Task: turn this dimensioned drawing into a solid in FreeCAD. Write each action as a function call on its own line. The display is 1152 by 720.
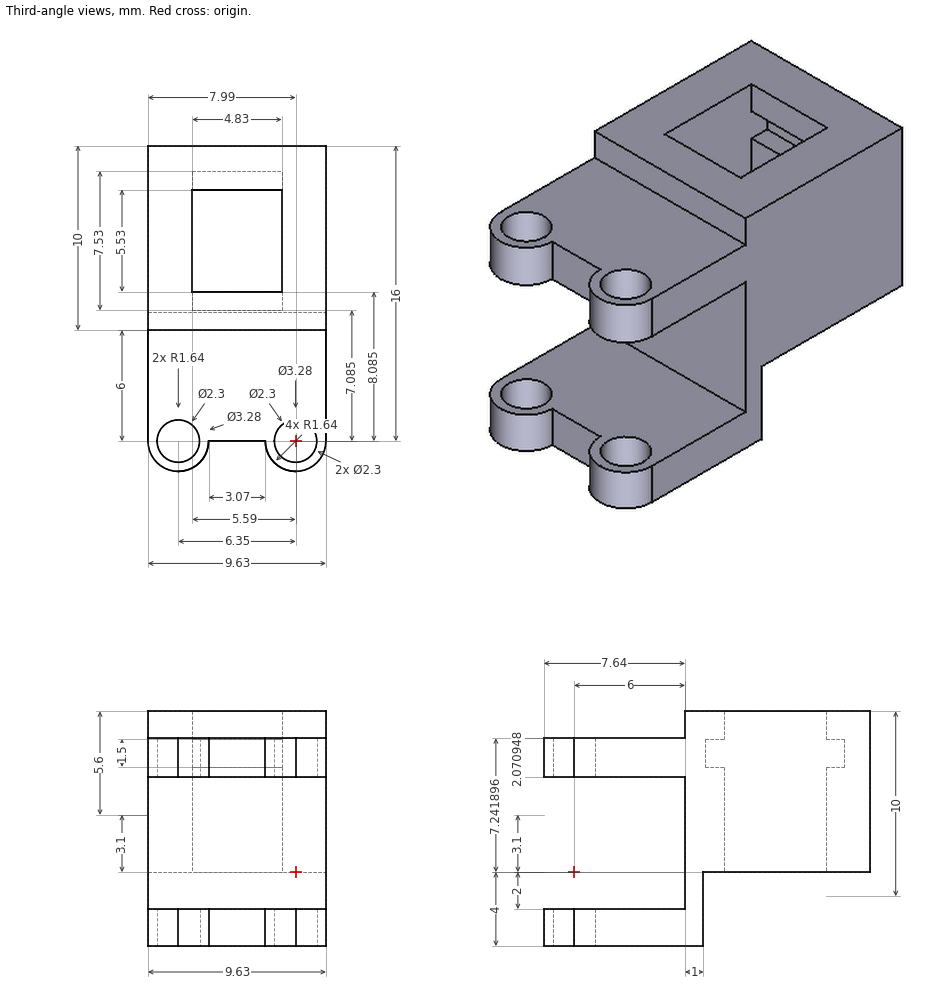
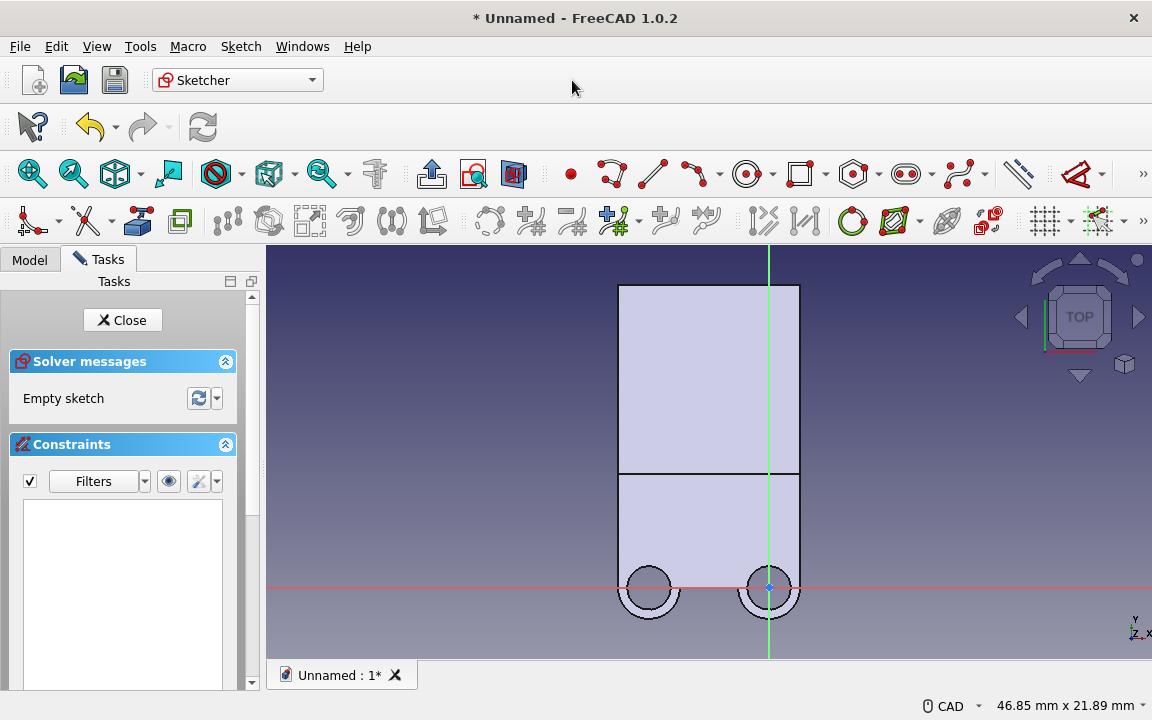
key(g)
key(r)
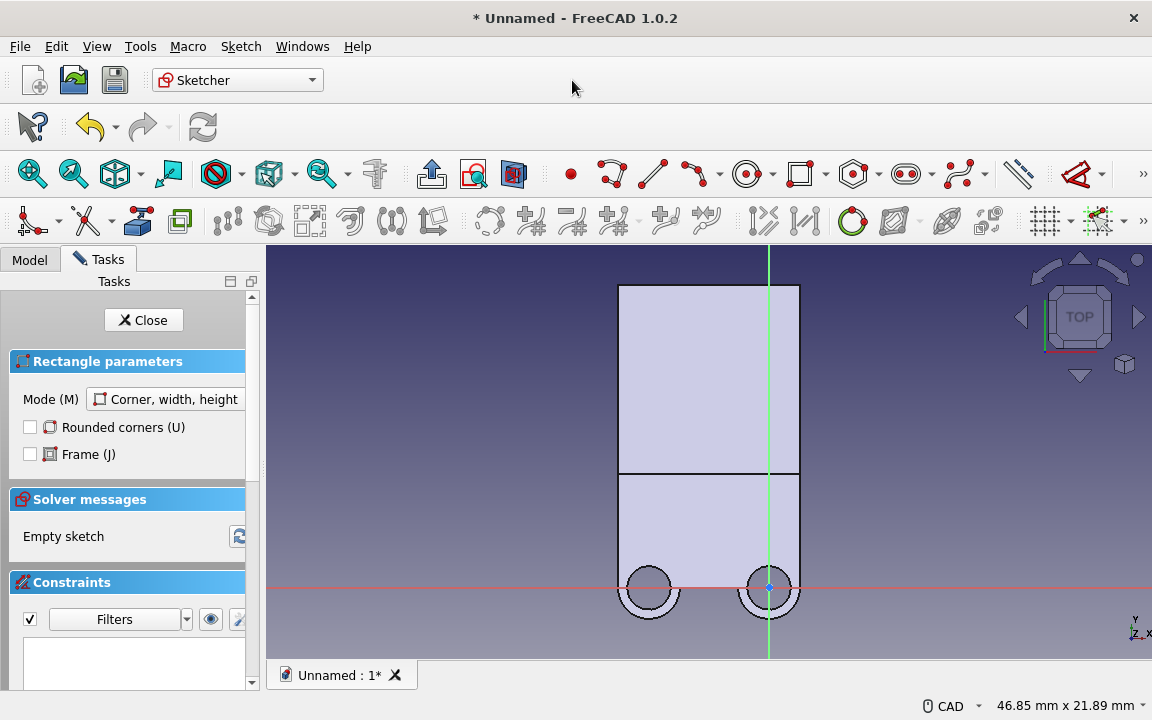
click(663, 330)
click(755, 435)
key(Escape)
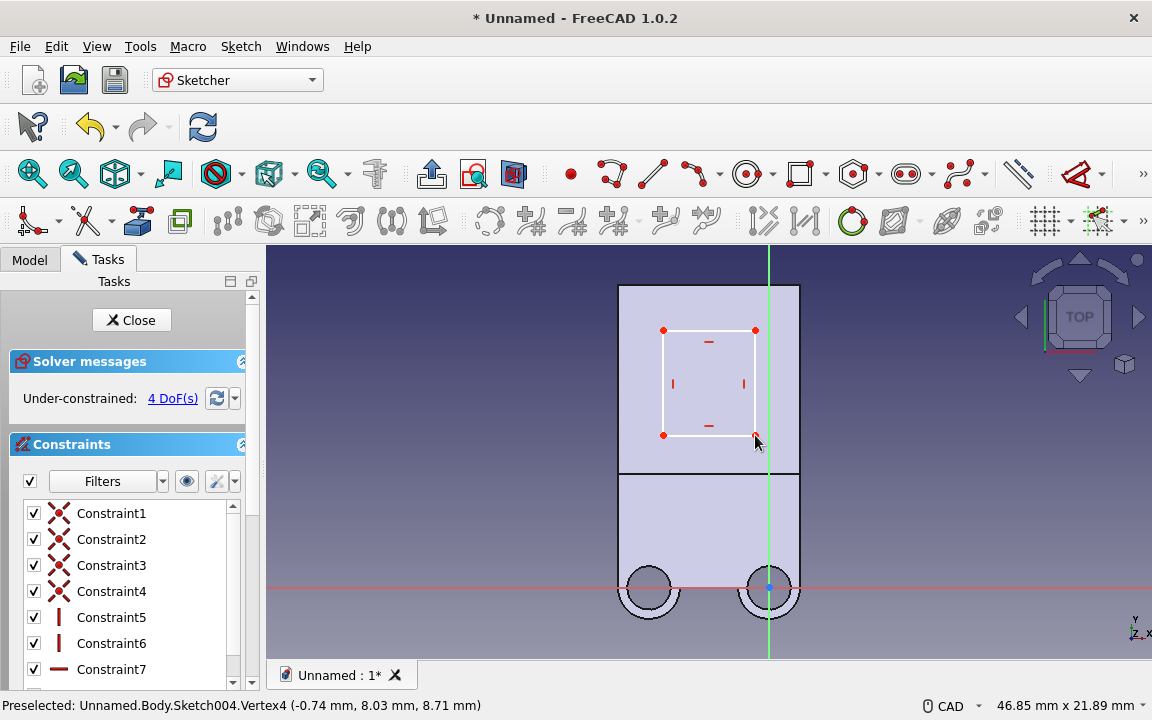
click(1076, 174)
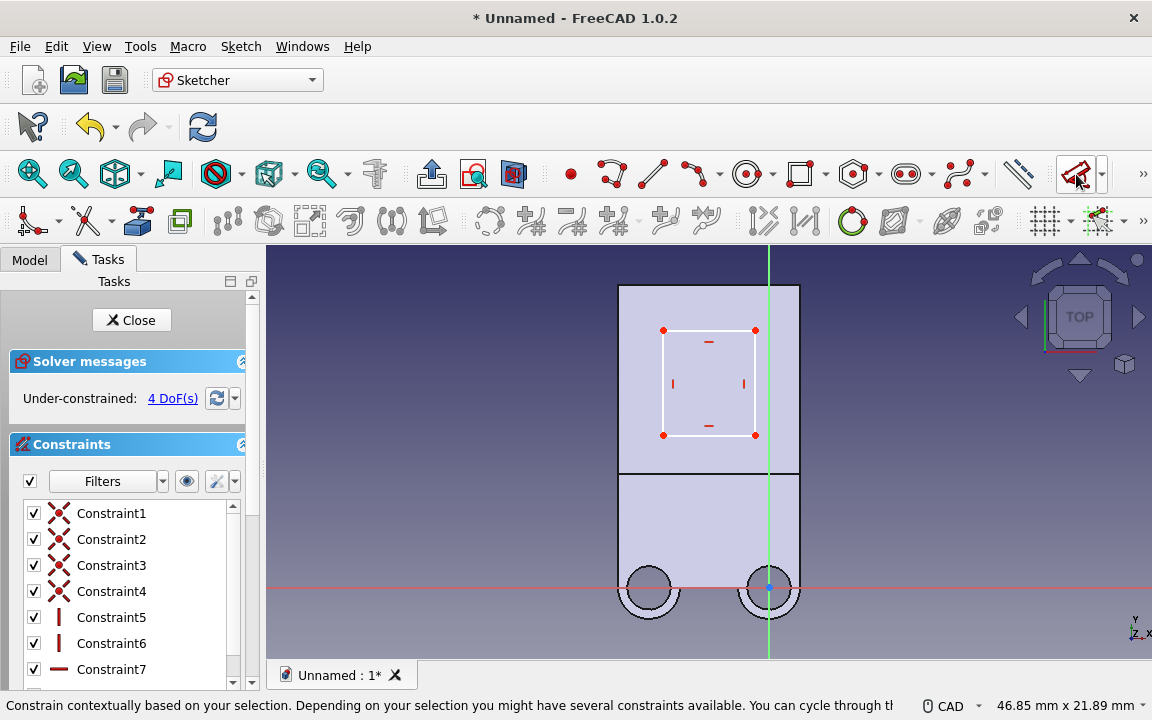
click(663, 363)
click(629, 384)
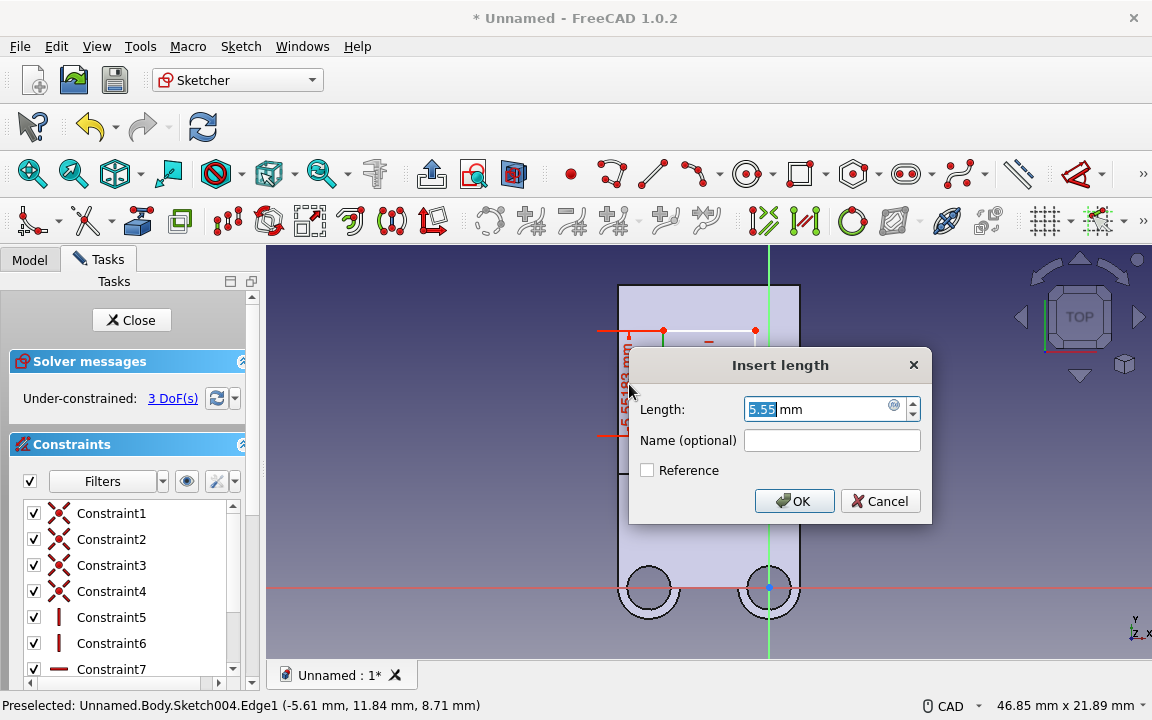
text(5.53)
key(Return)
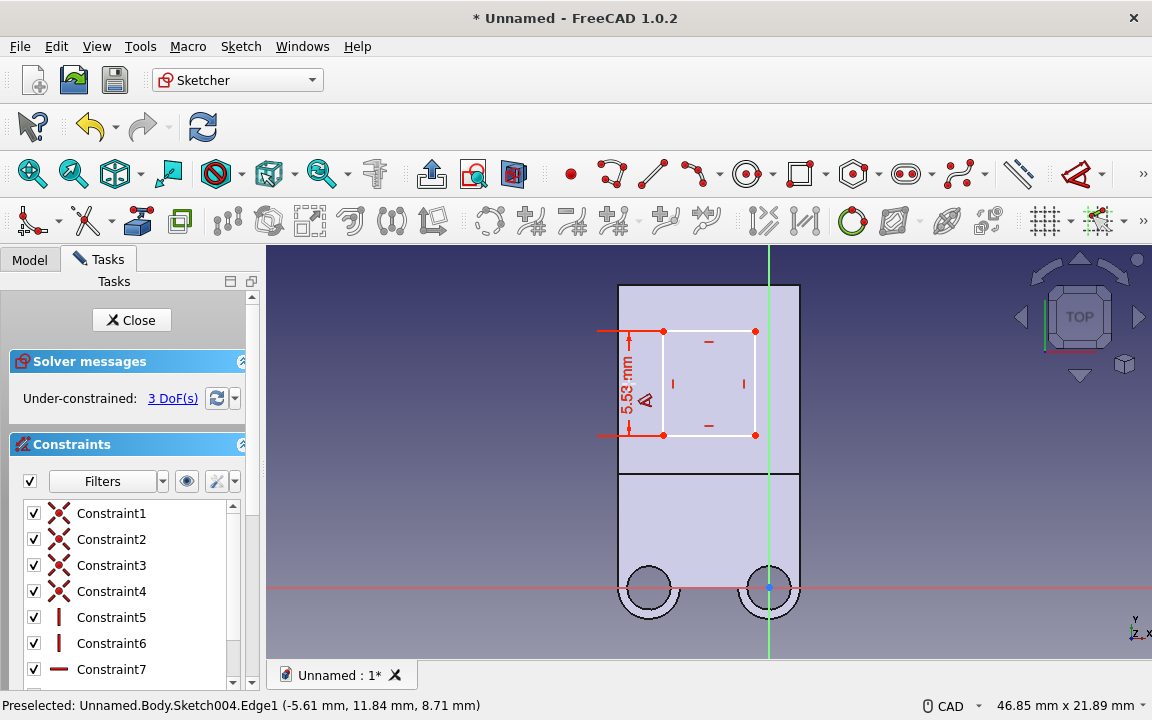
click(691, 436)
click(709, 402)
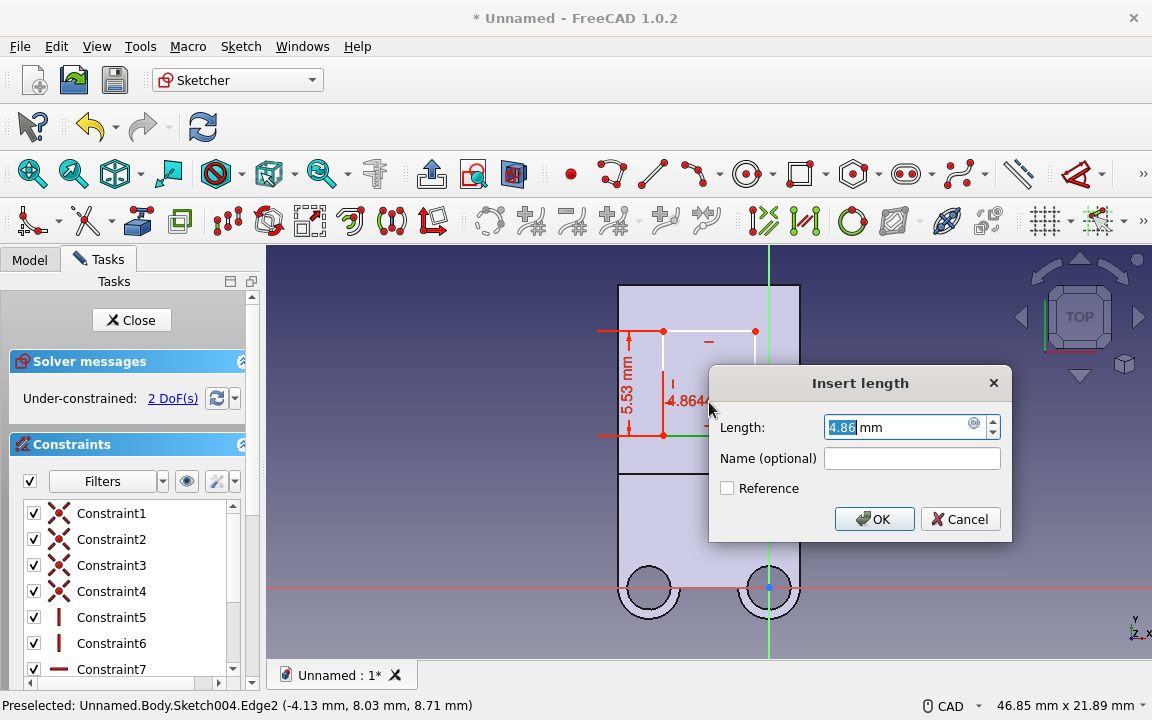
text(4.83)
key(Return)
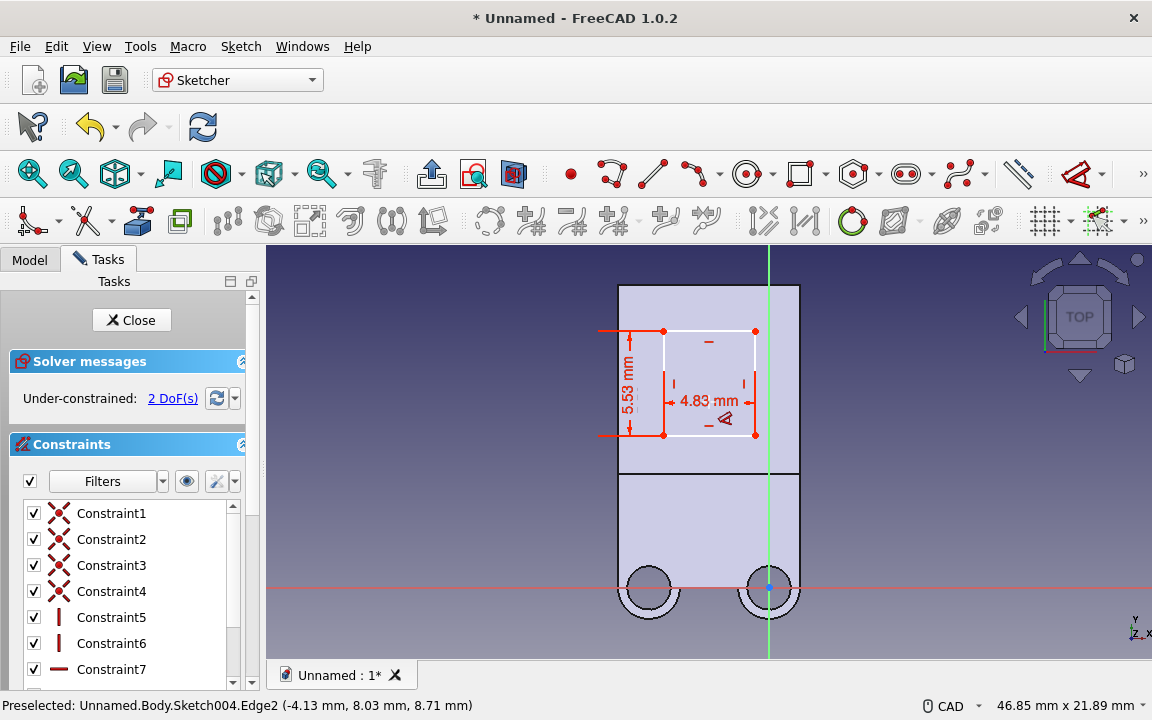
click(664, 331)
click(716, 622)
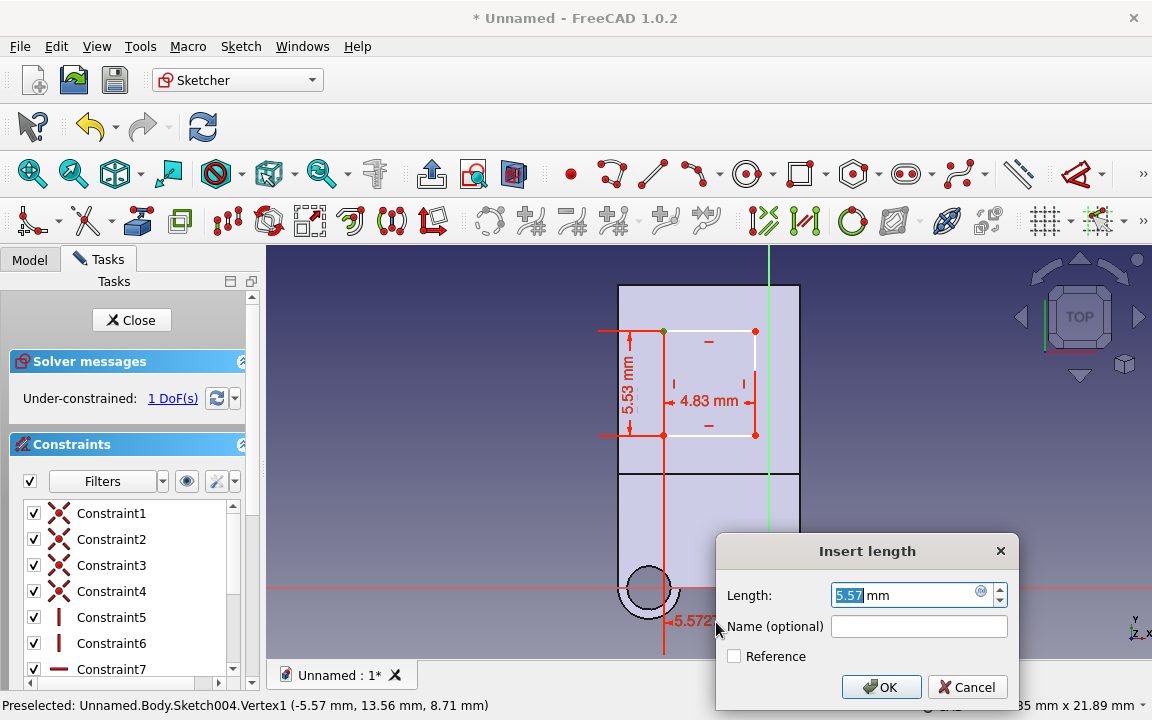
text(5.59)
key(Return)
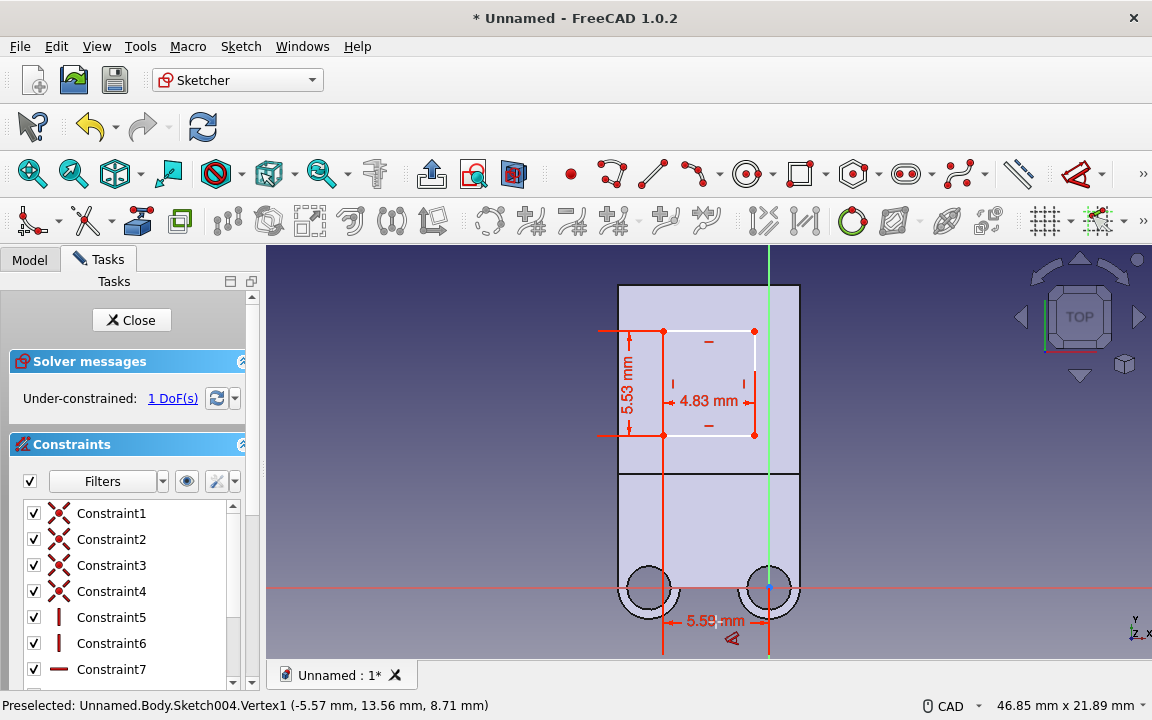
click(663, 436)
click(803, 512)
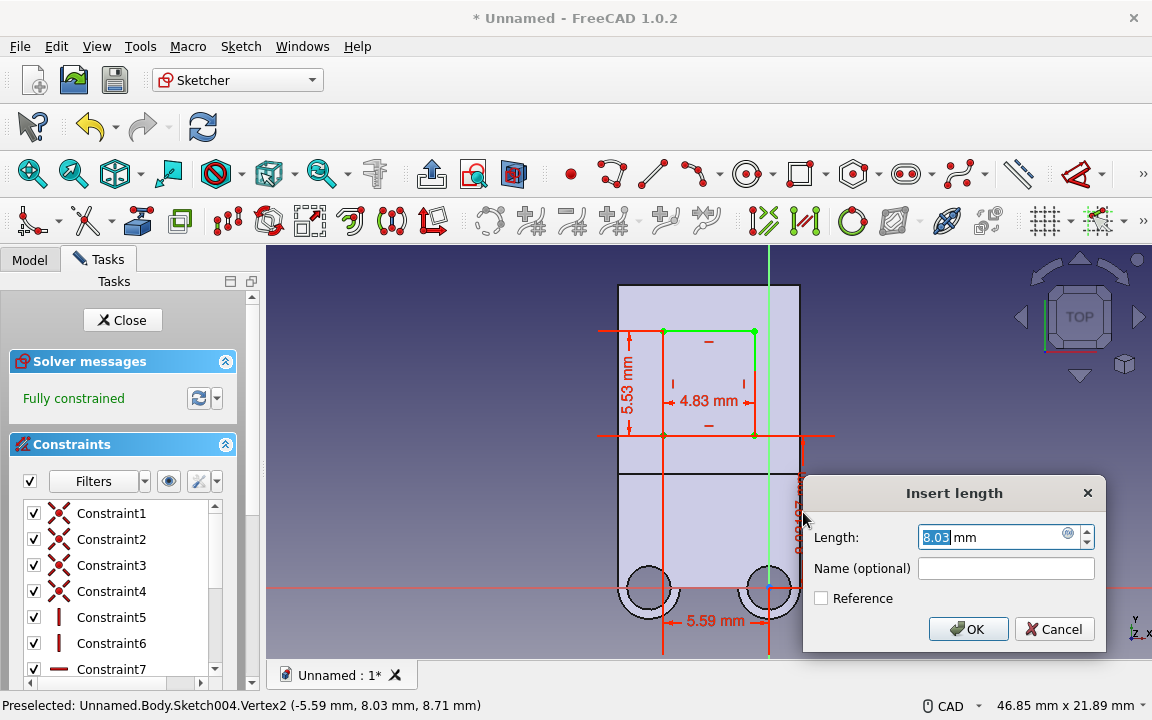
text(8.085)
key(Return)
key(Escape)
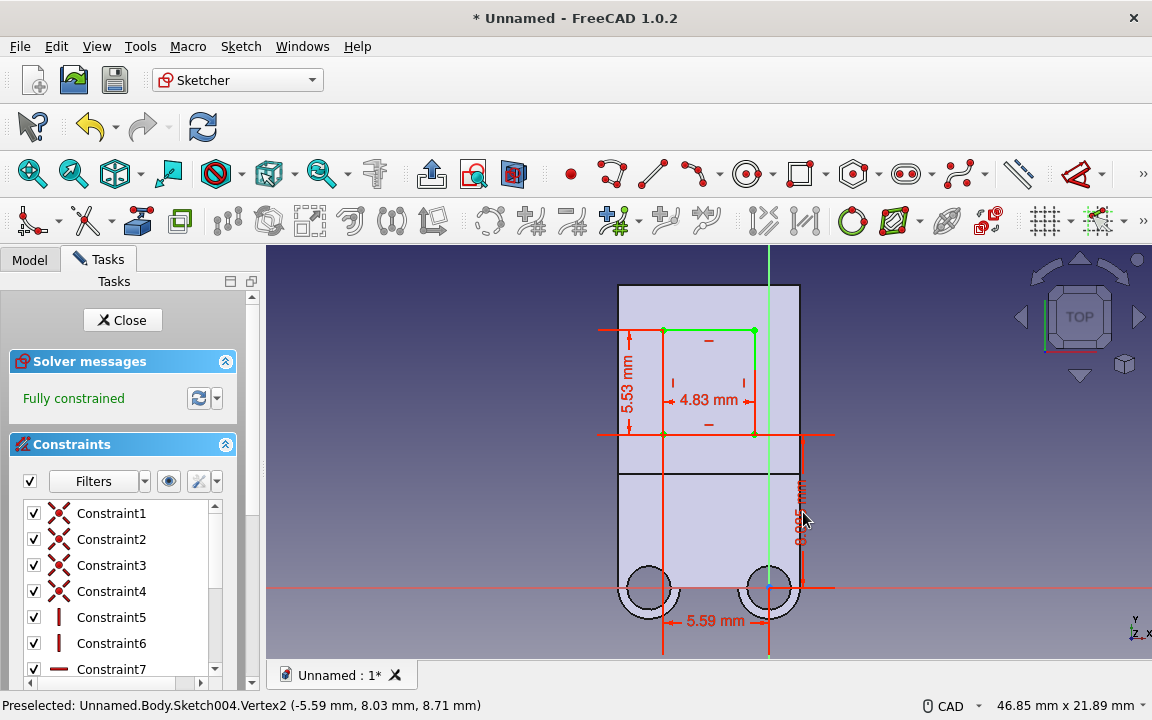
click(123, 320)